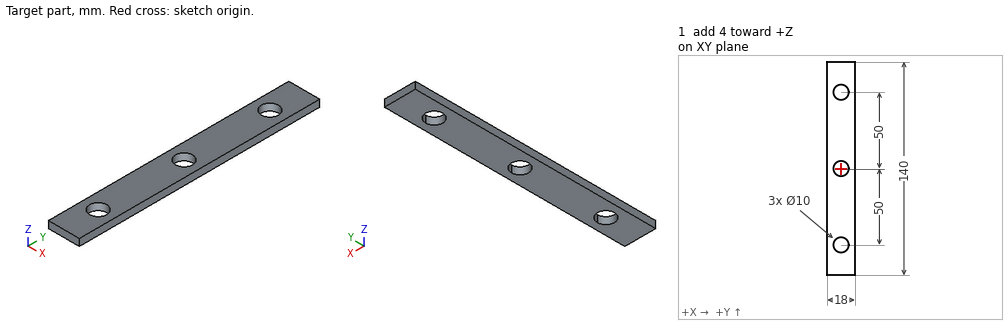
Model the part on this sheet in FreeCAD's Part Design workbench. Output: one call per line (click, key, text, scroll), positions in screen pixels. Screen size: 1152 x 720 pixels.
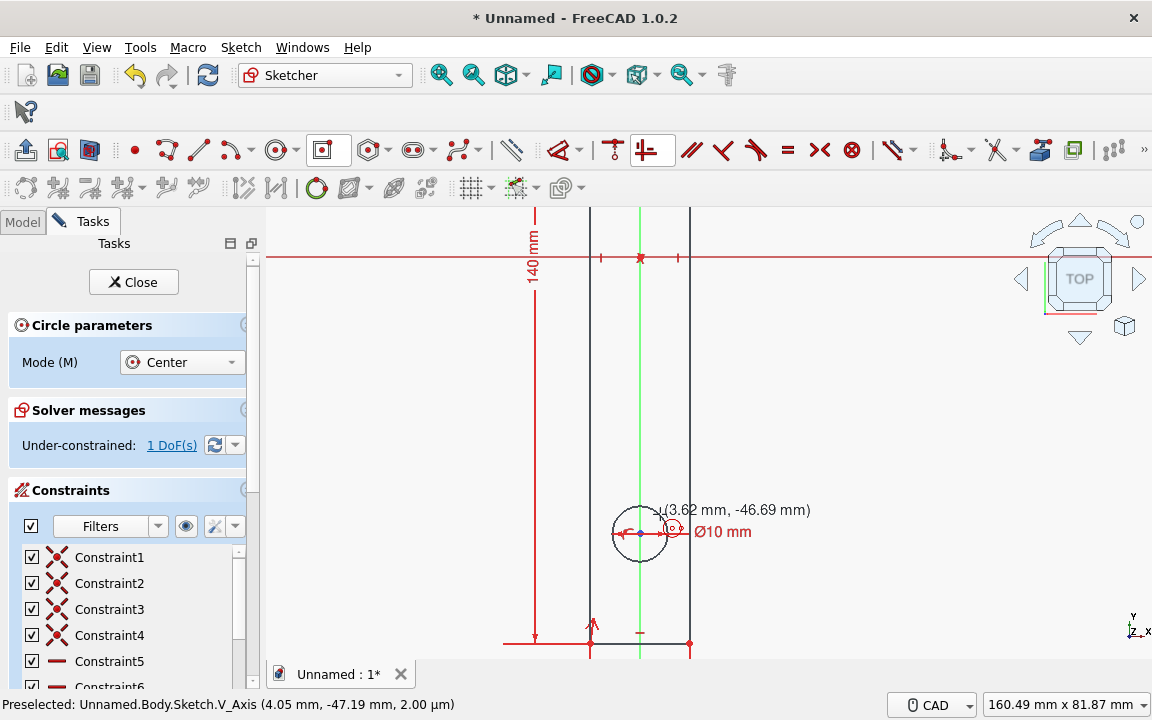
click(640, 257)
move(660, 238)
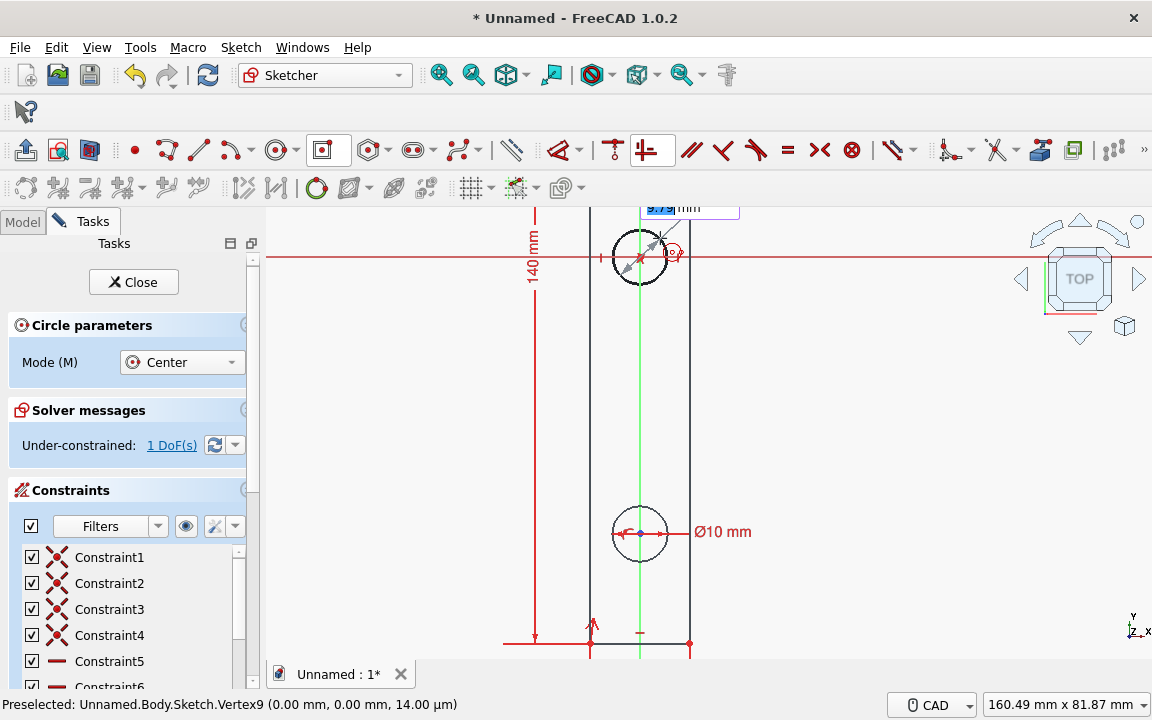
text(10)
key(Return)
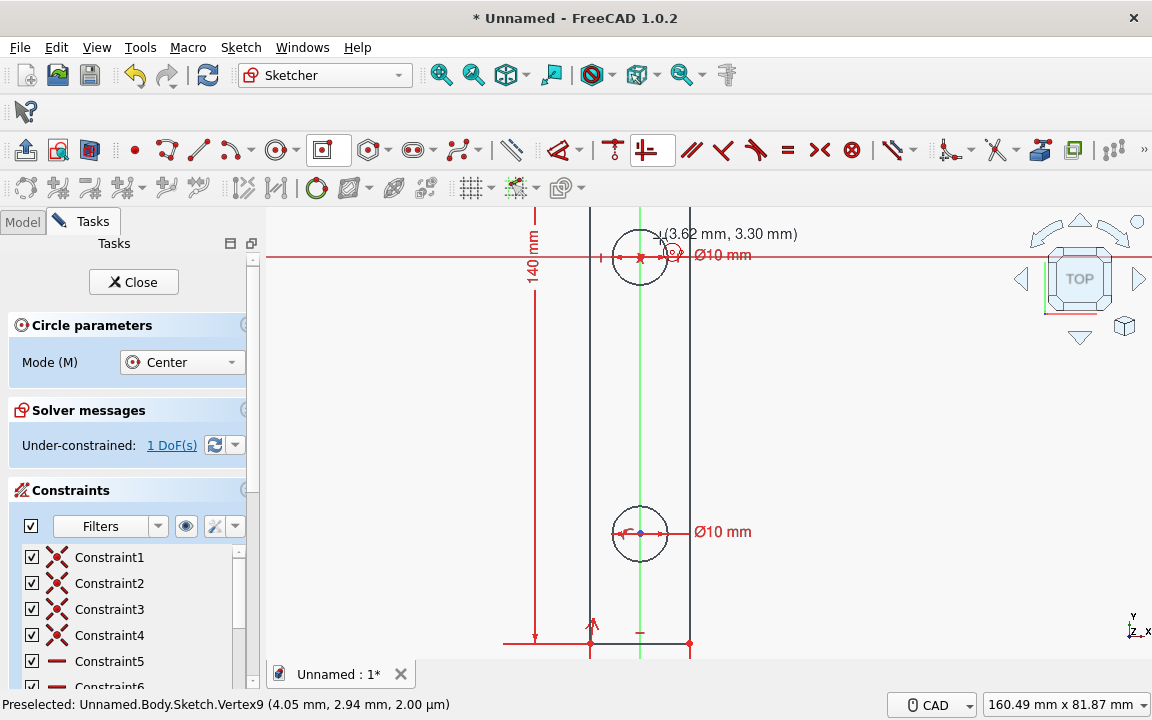
scroll(641, 535, down, 5)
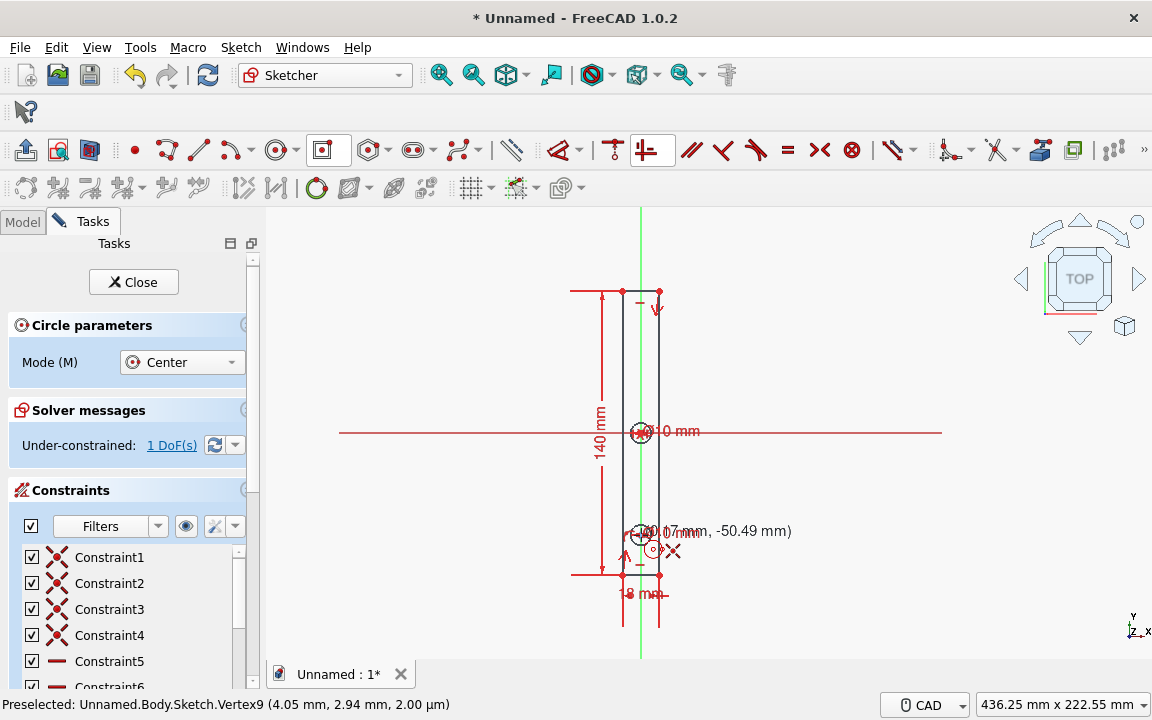
scroll(641, 332, up, 5)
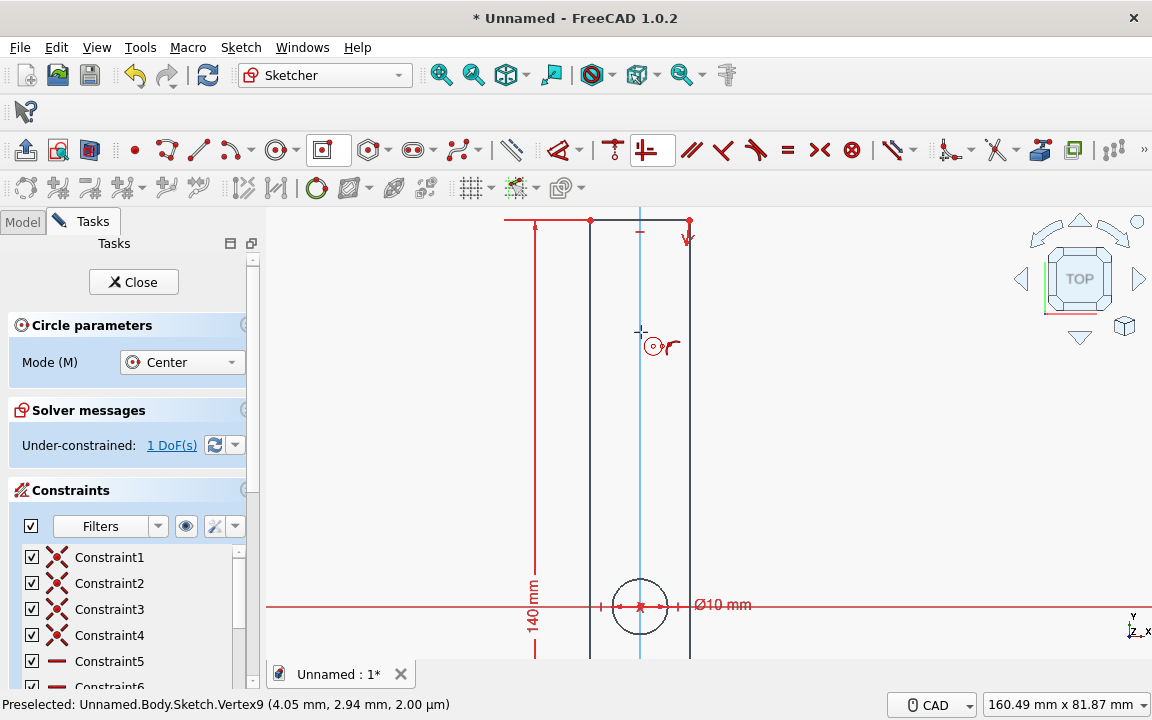
click(640, 331)
move(660, 311)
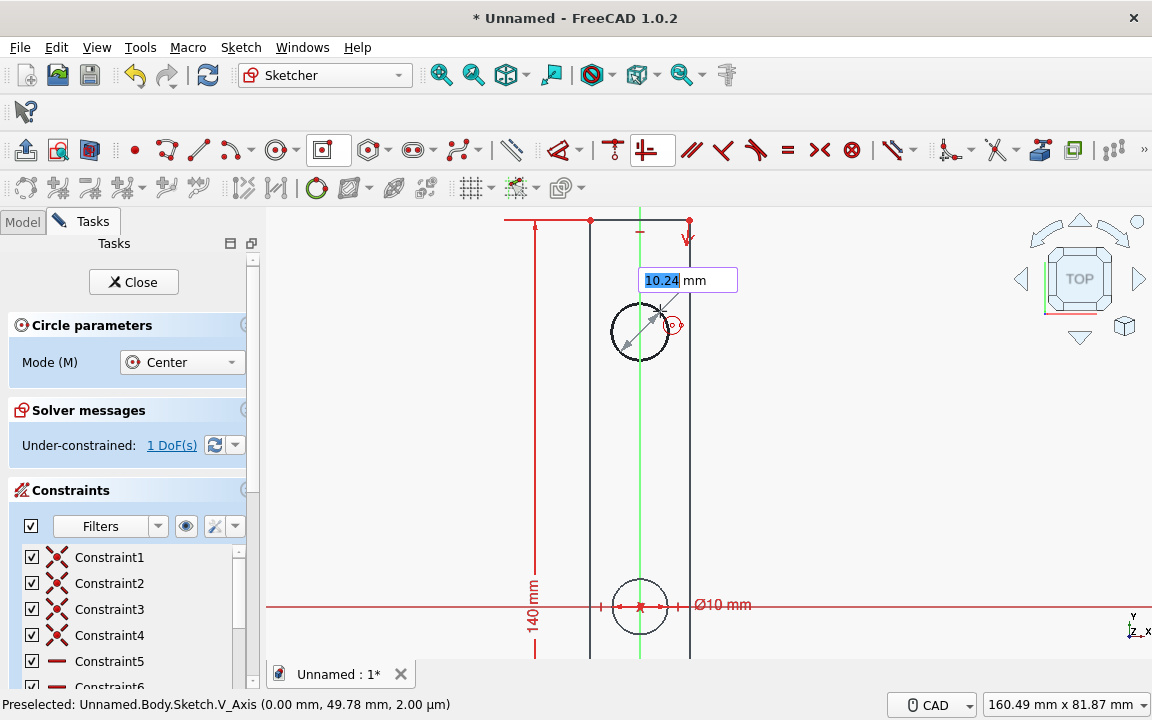
text(10)
key(Return)
key(Escape)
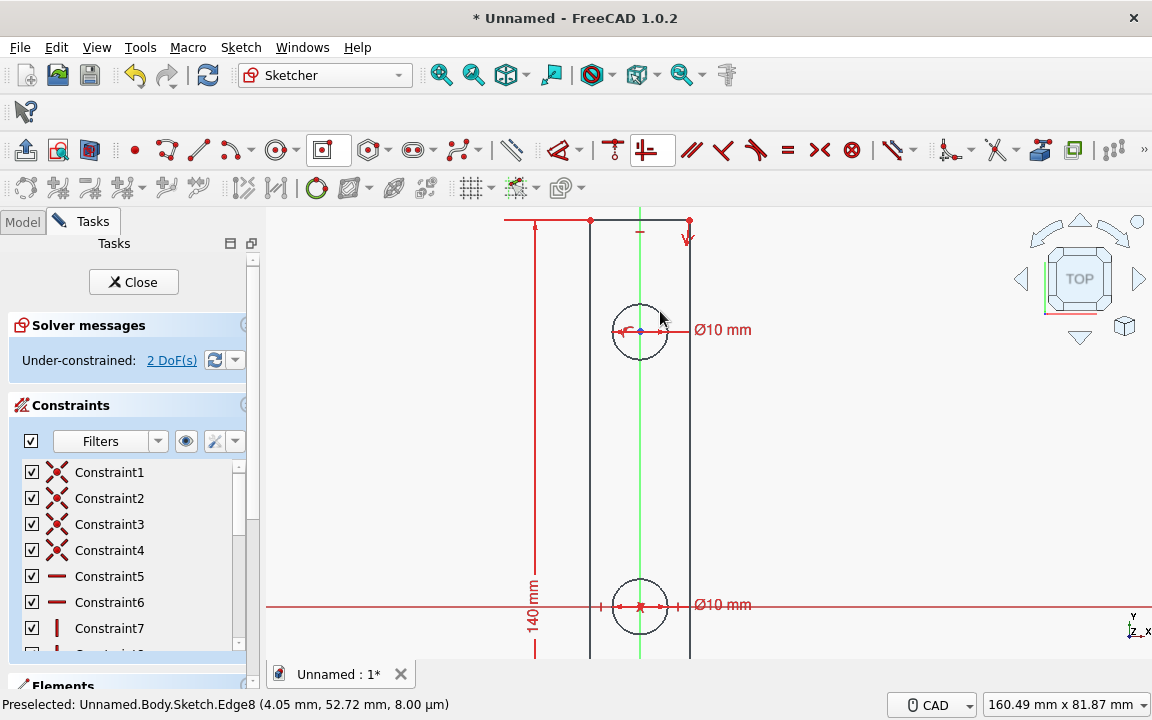
click(558, 150)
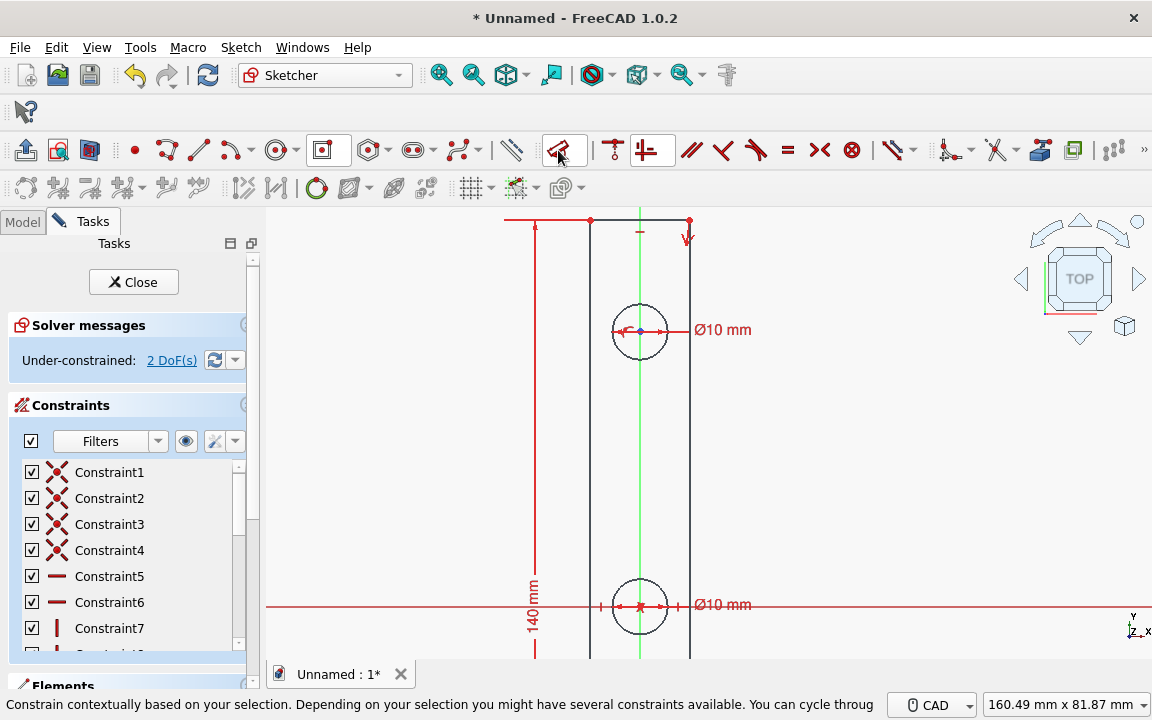
scroll(641, 332, down, 5)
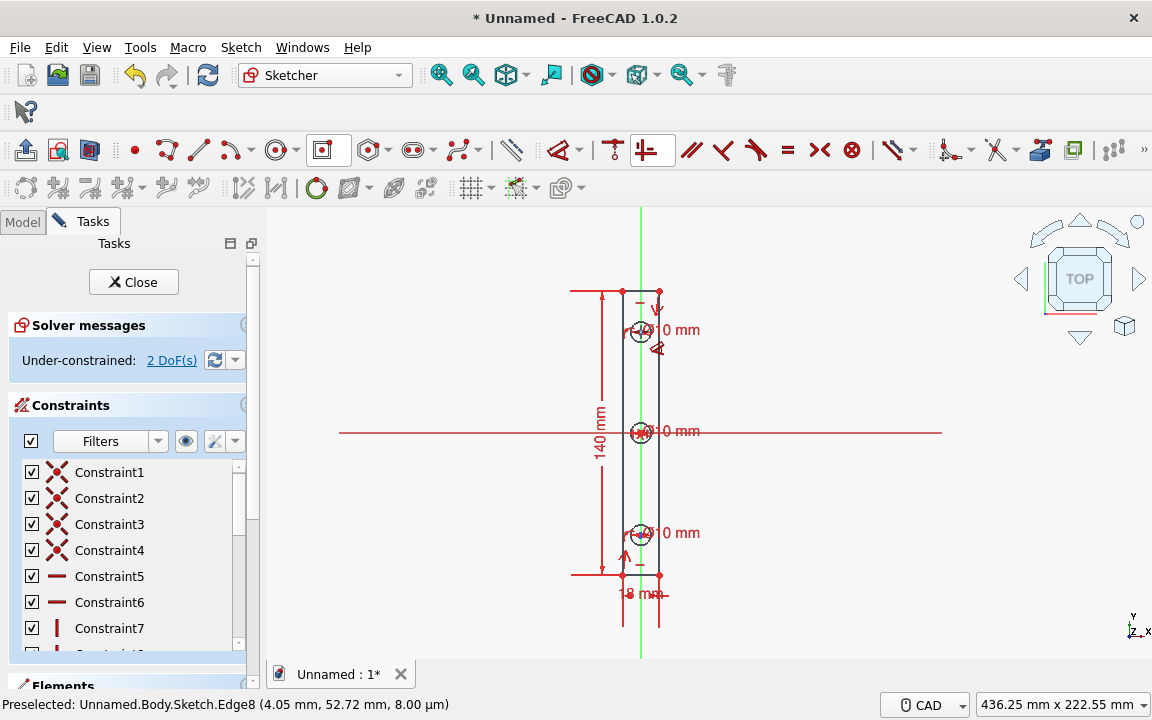
click(641, 535)
click(675, 484)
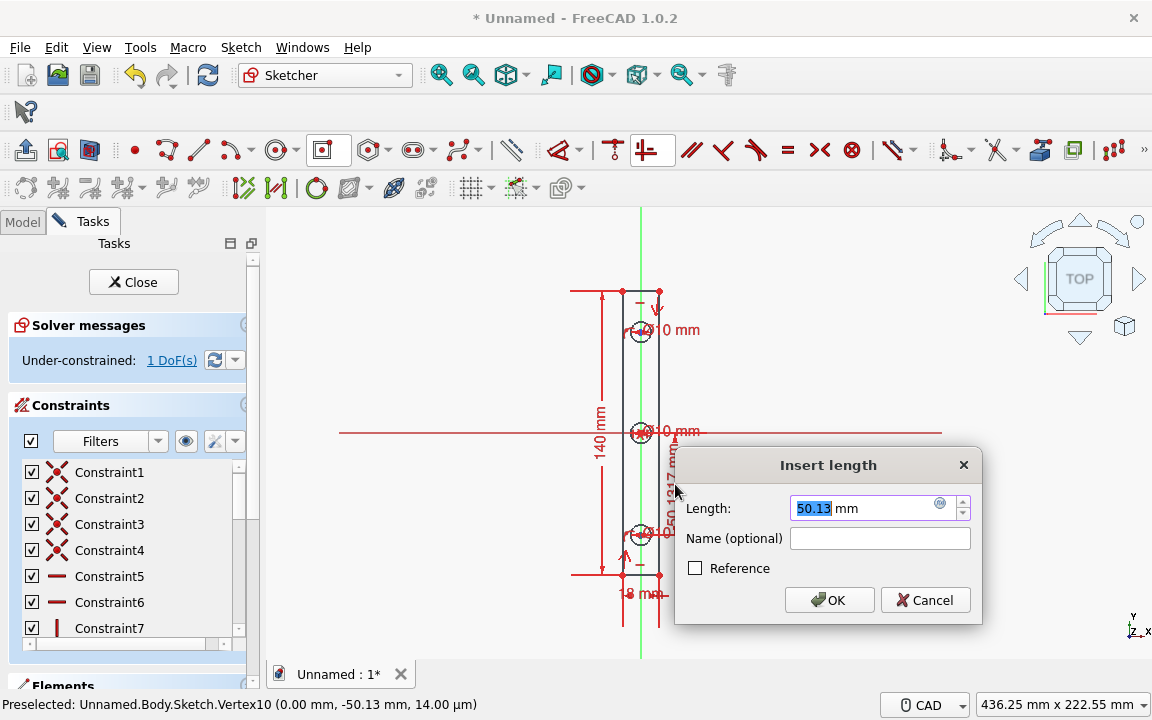
text(50)
key(Return)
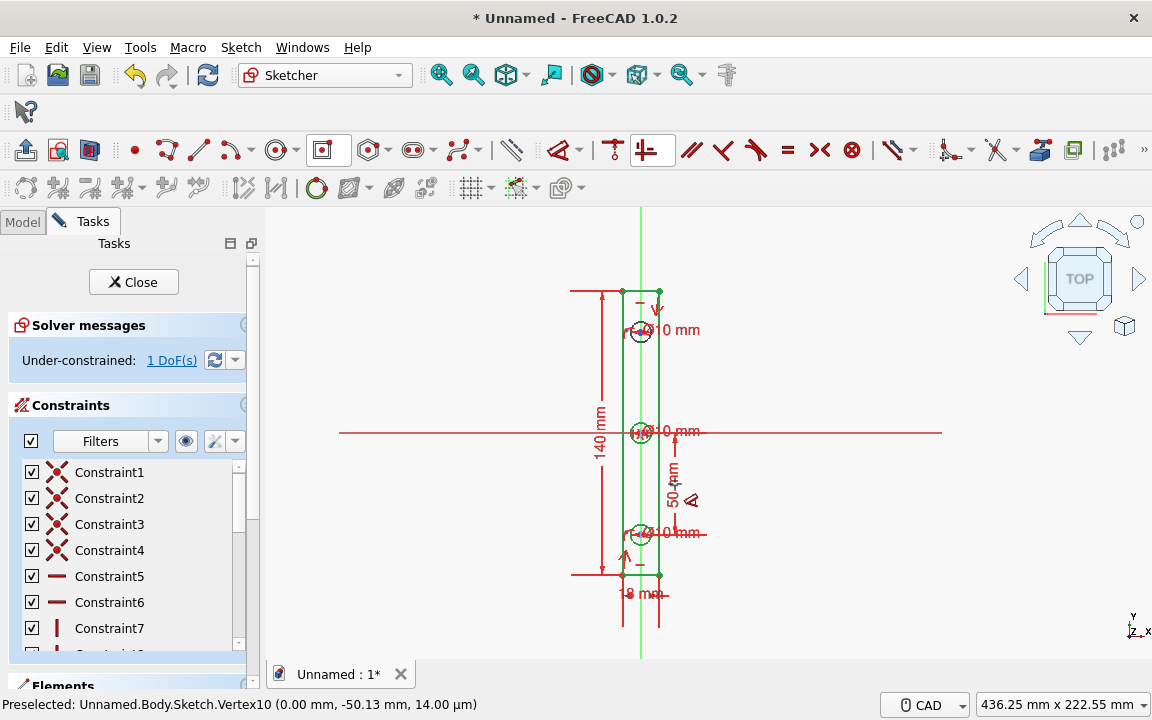
click(641, 332)
click(675, 383)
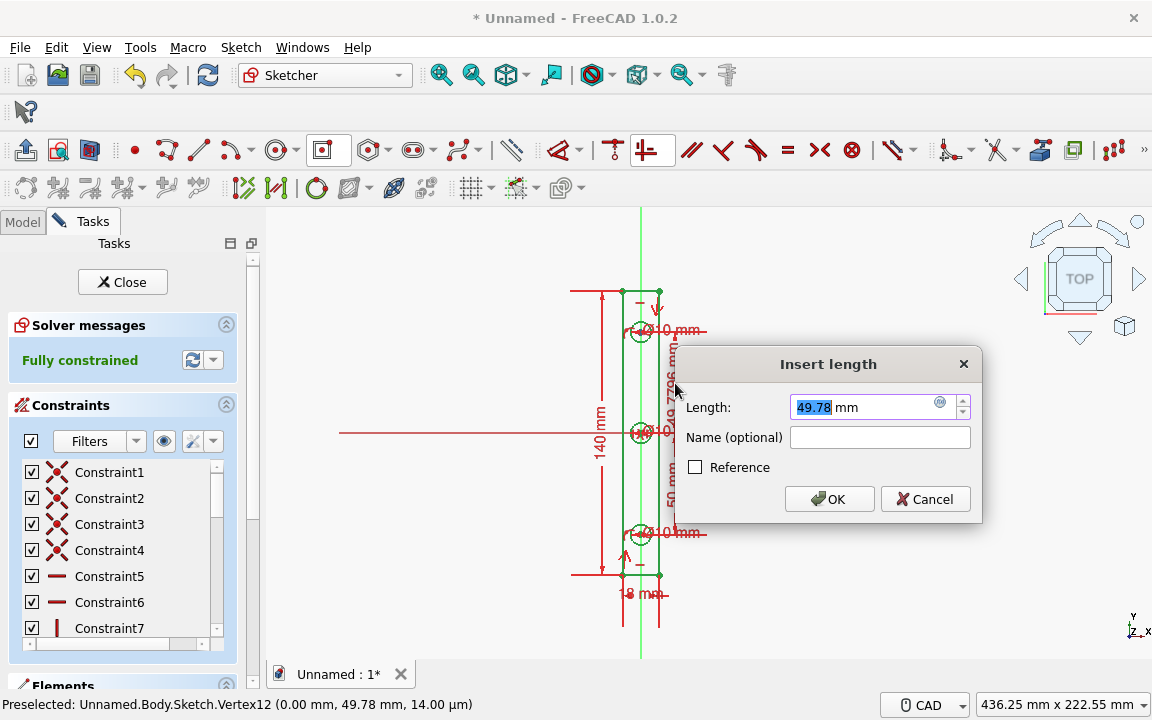
text(50)
key(Return)
key(Escape)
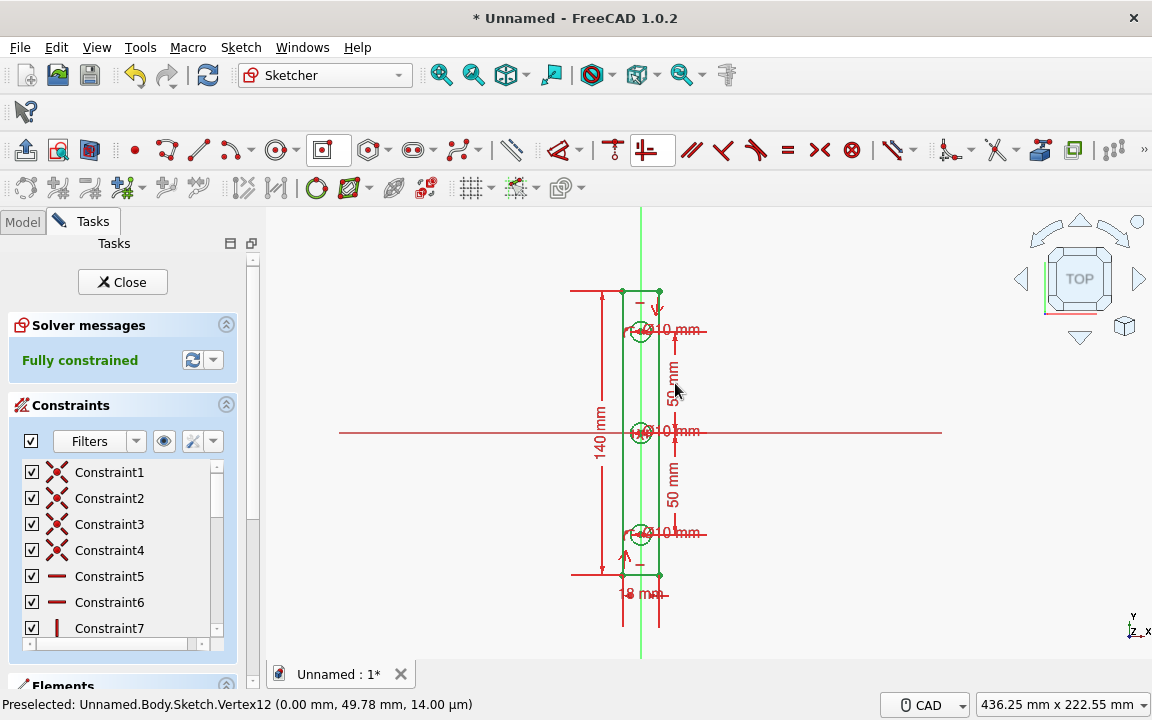
click(123, 282)